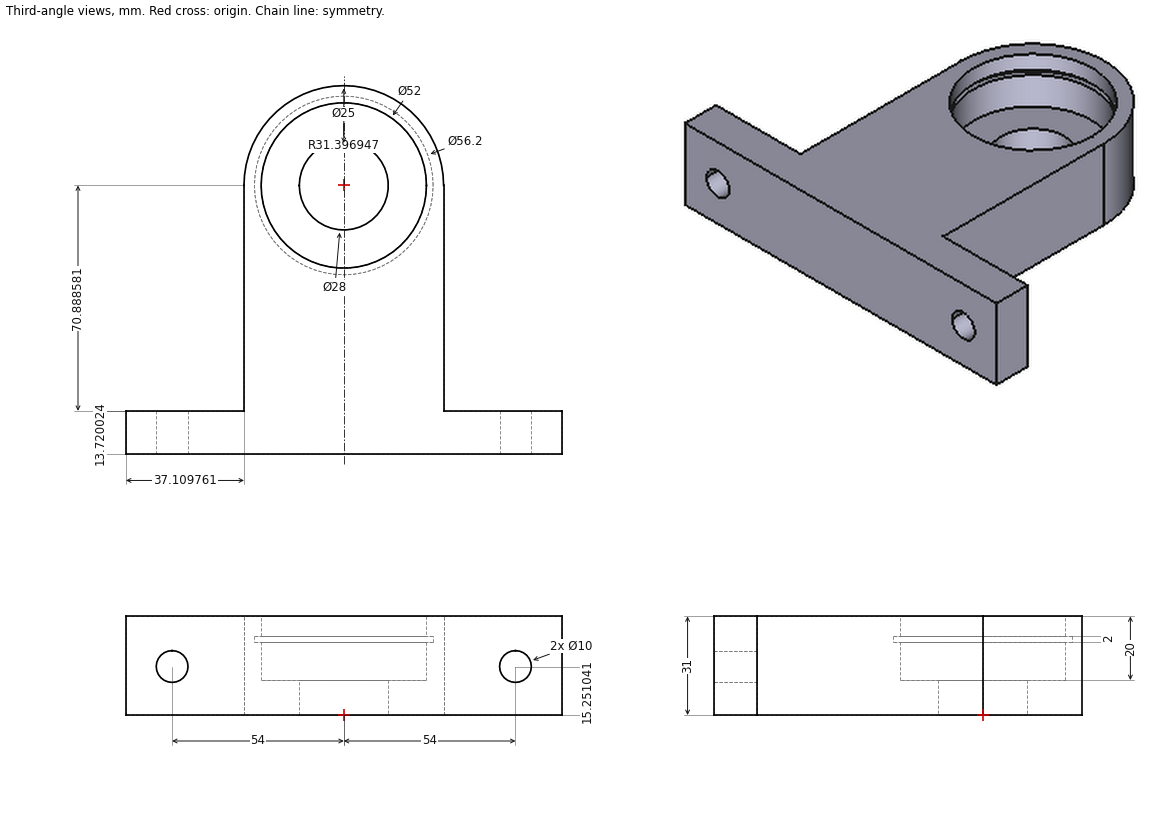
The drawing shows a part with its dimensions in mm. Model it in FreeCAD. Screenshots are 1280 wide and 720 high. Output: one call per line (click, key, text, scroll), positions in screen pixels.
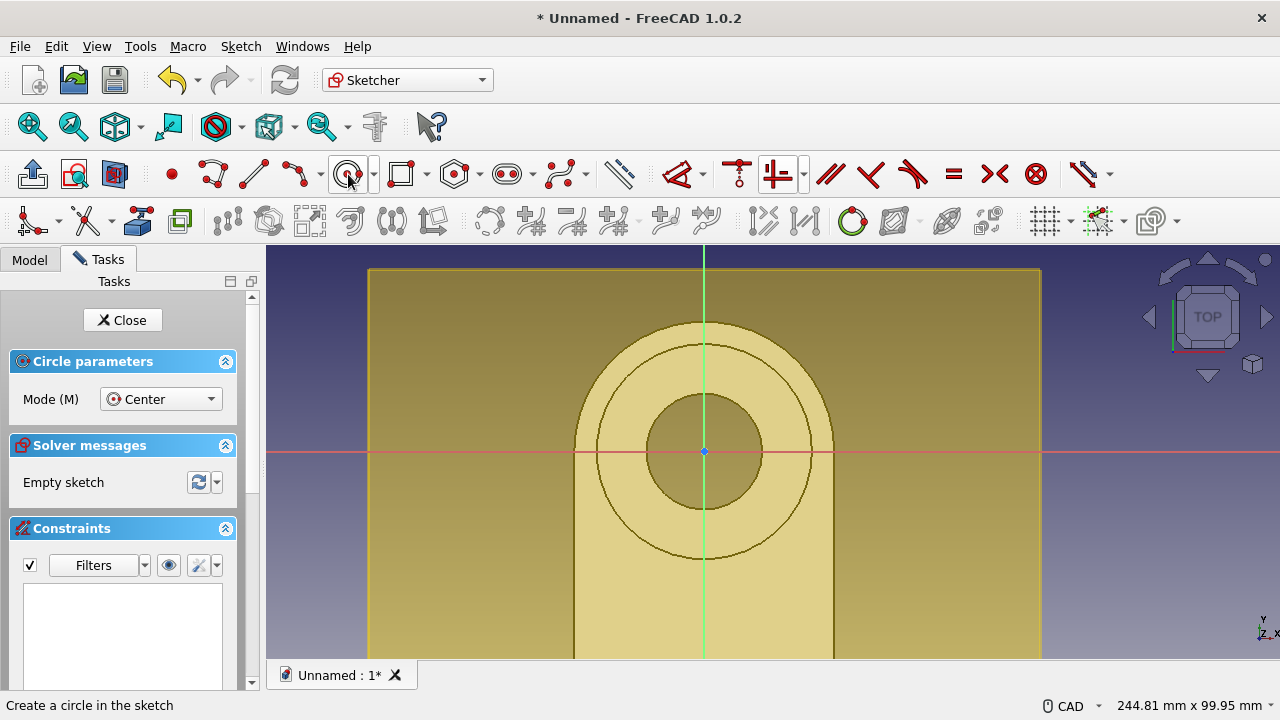
click(704, 452)
click(787, 369)
key(Escape)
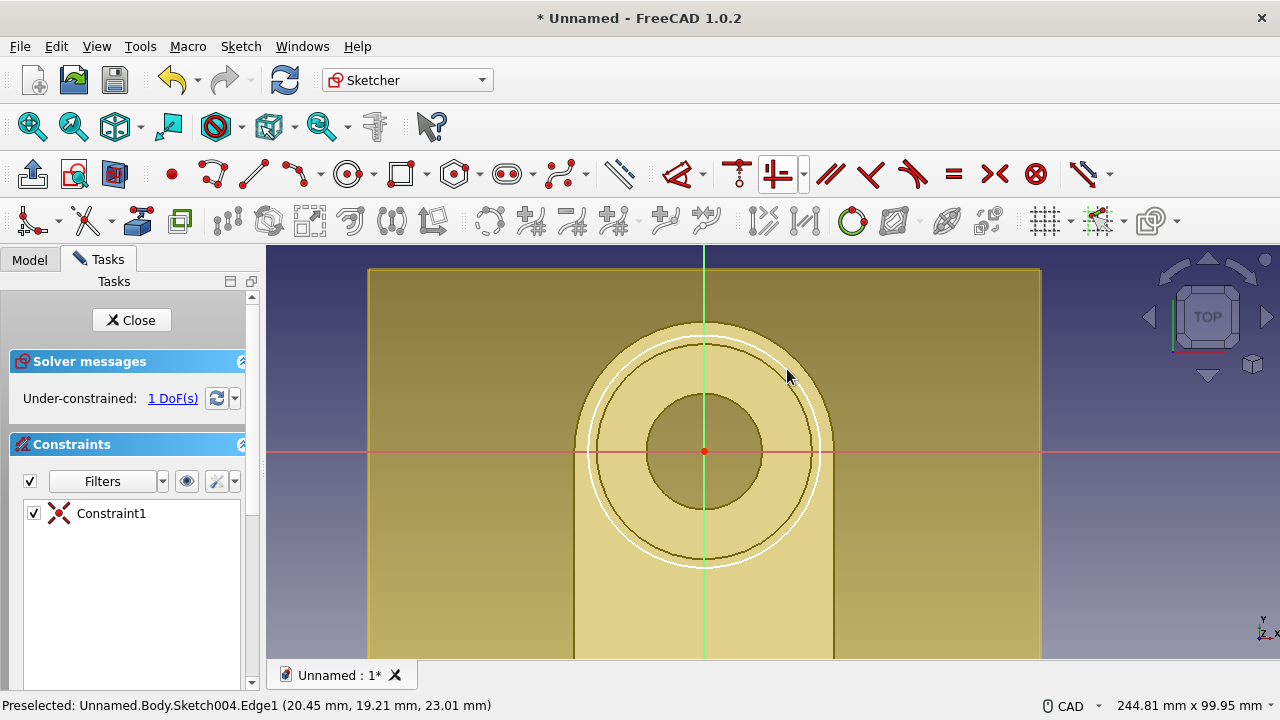
key(d)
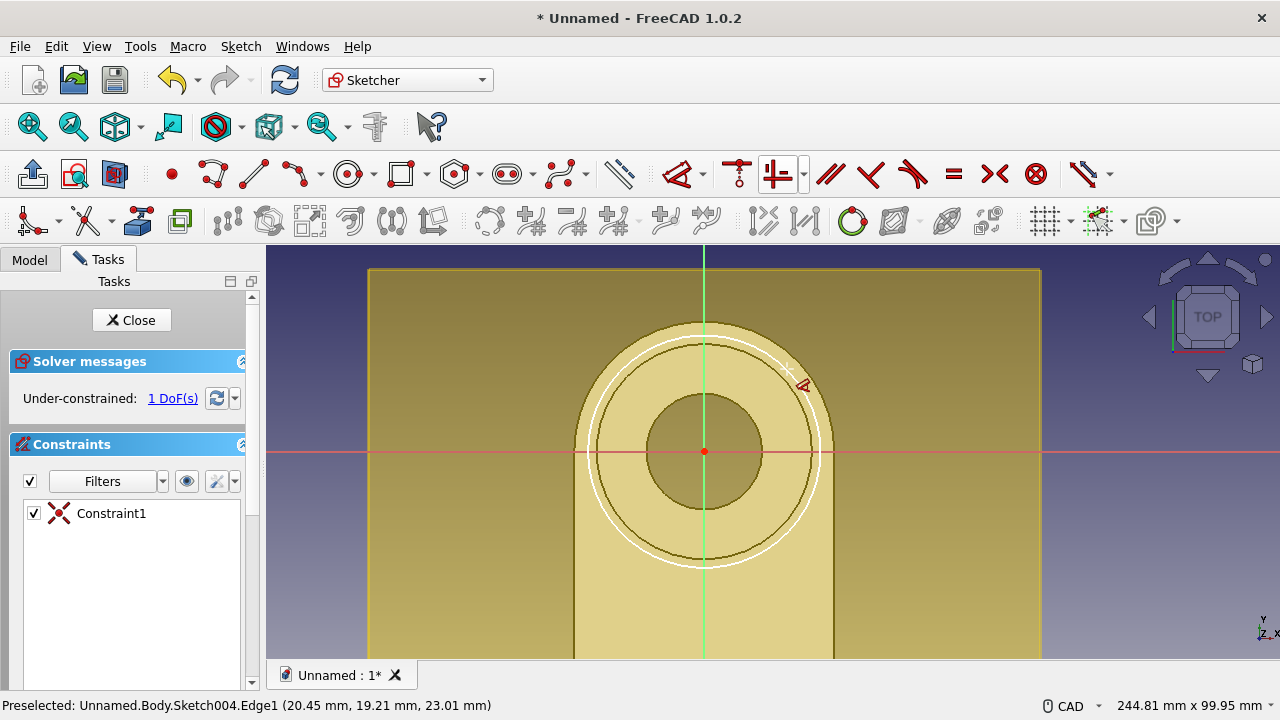
click(786, 369)
click(808, 346)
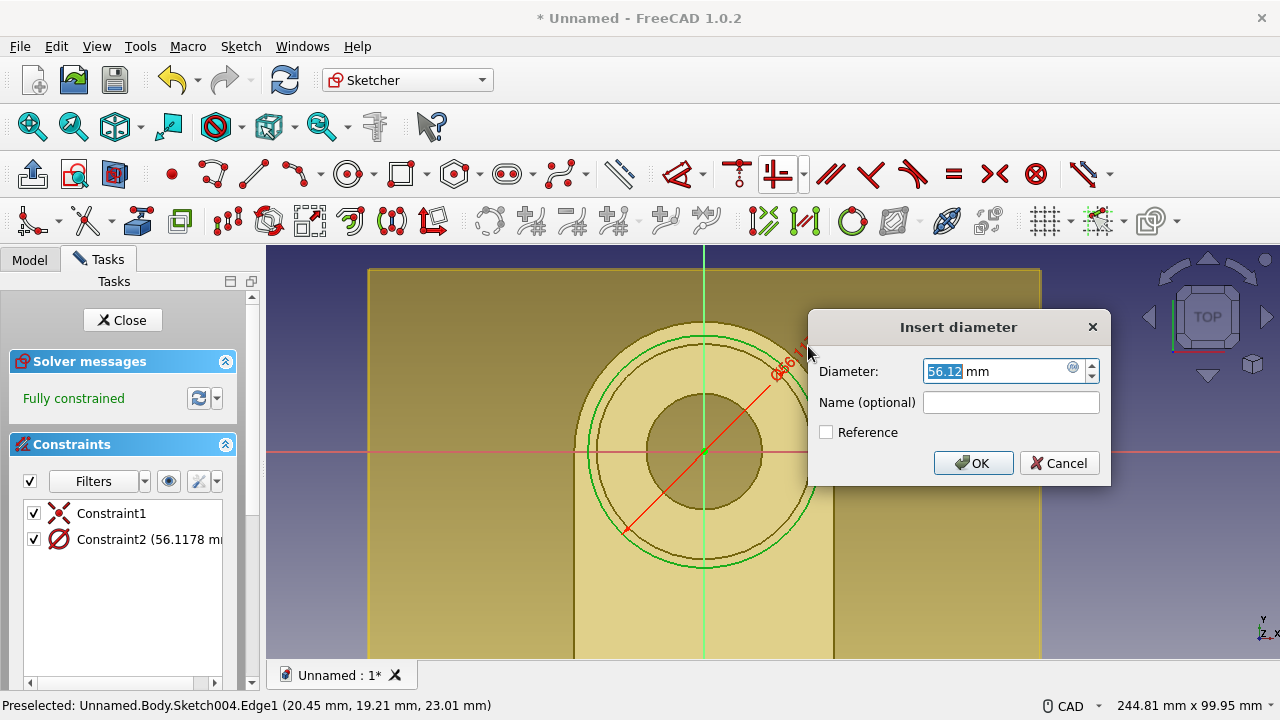
text(56.2)
key(Return)
key(Escape)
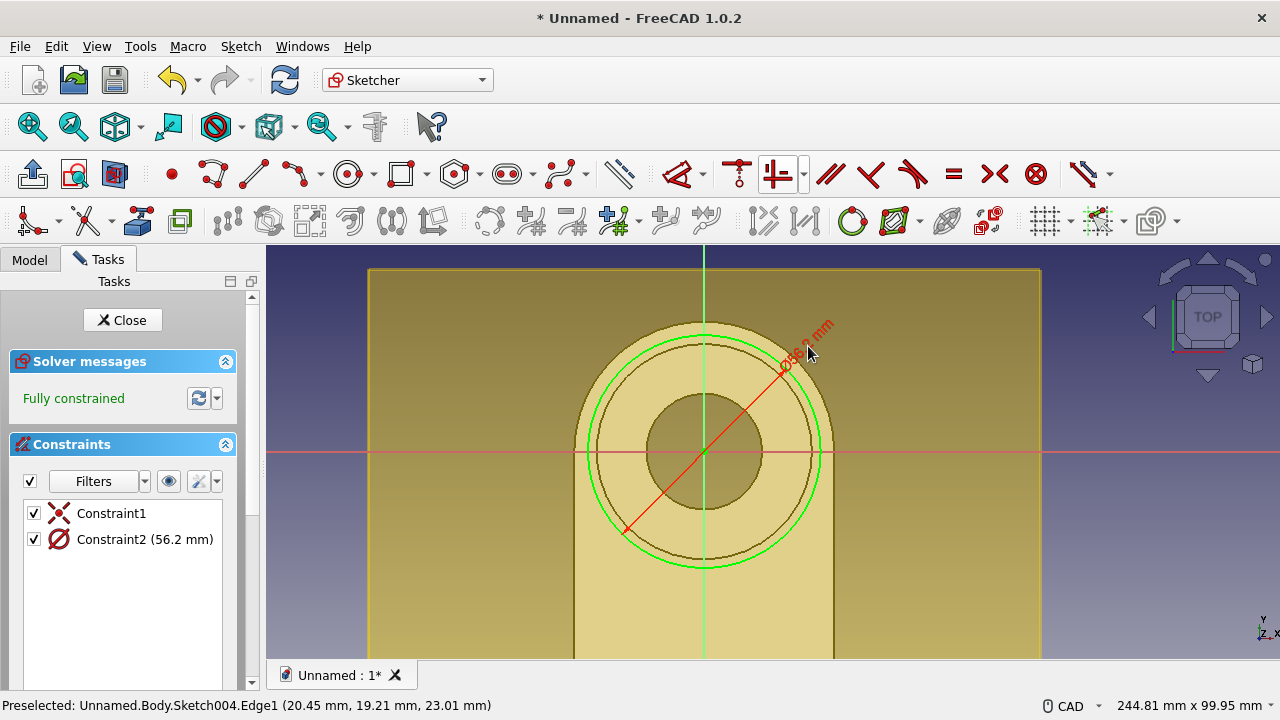
click(123, 320)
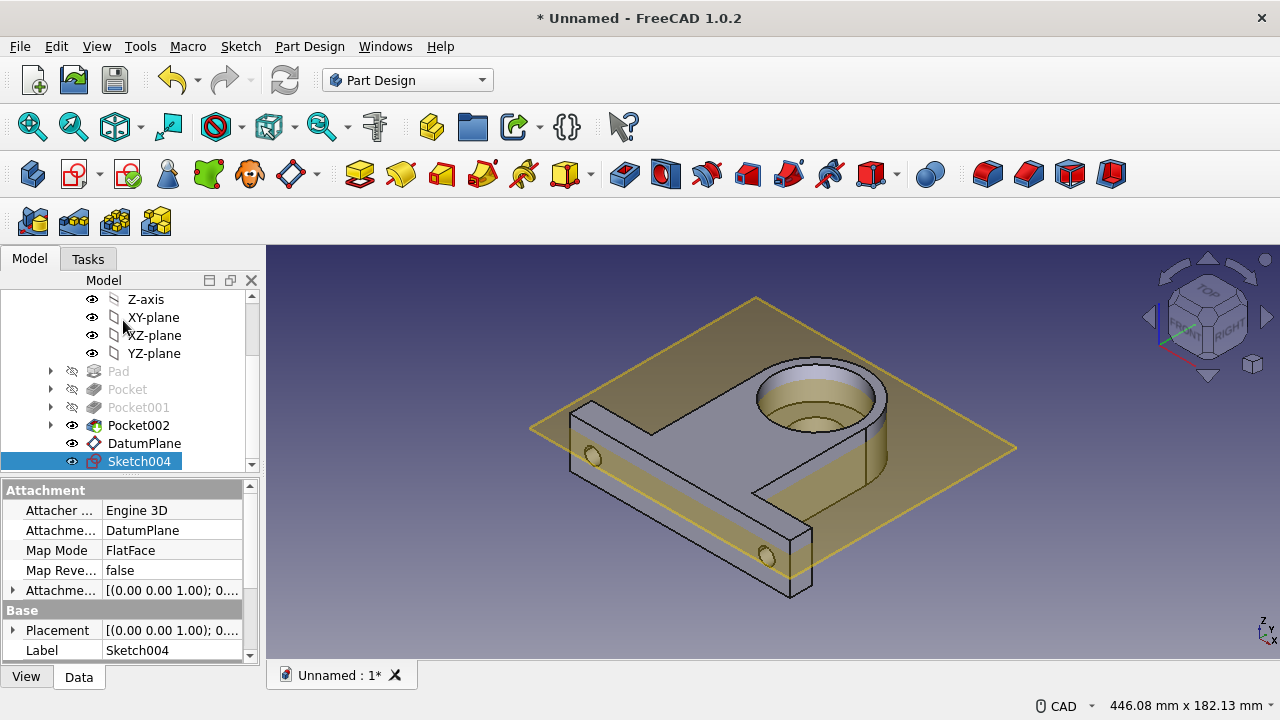
click(625, 174)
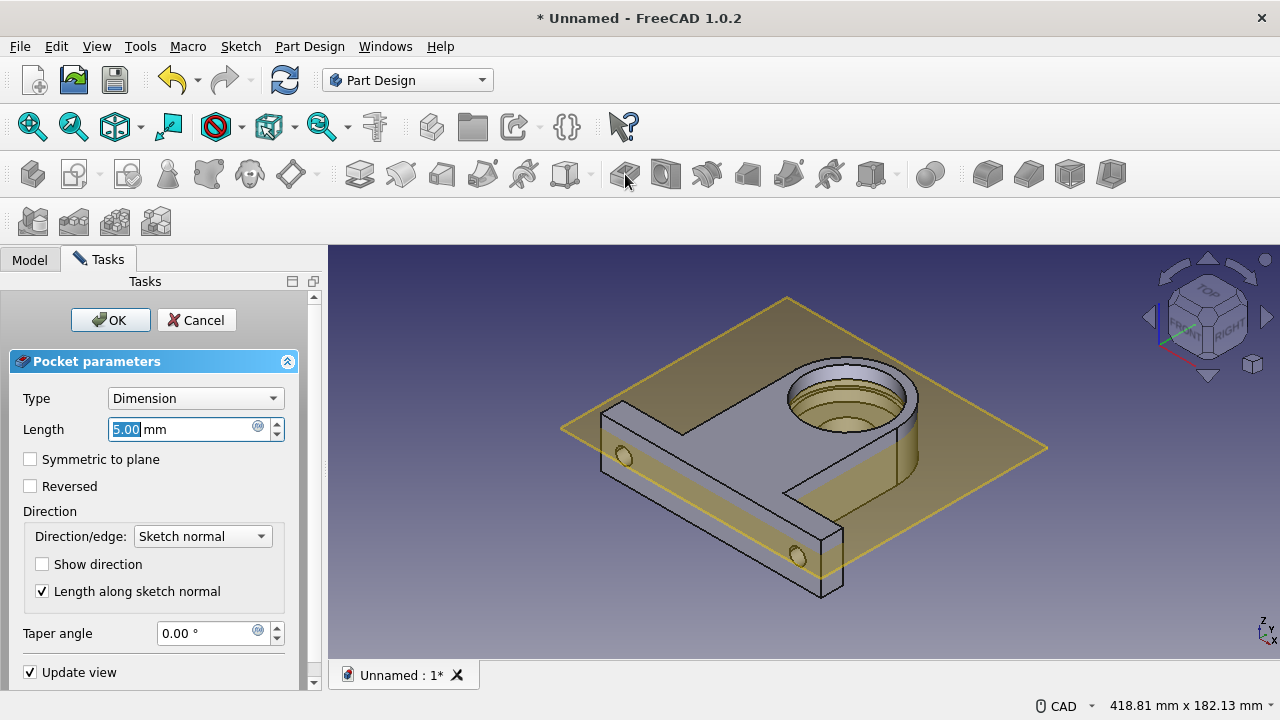
text(2)
key(Tab)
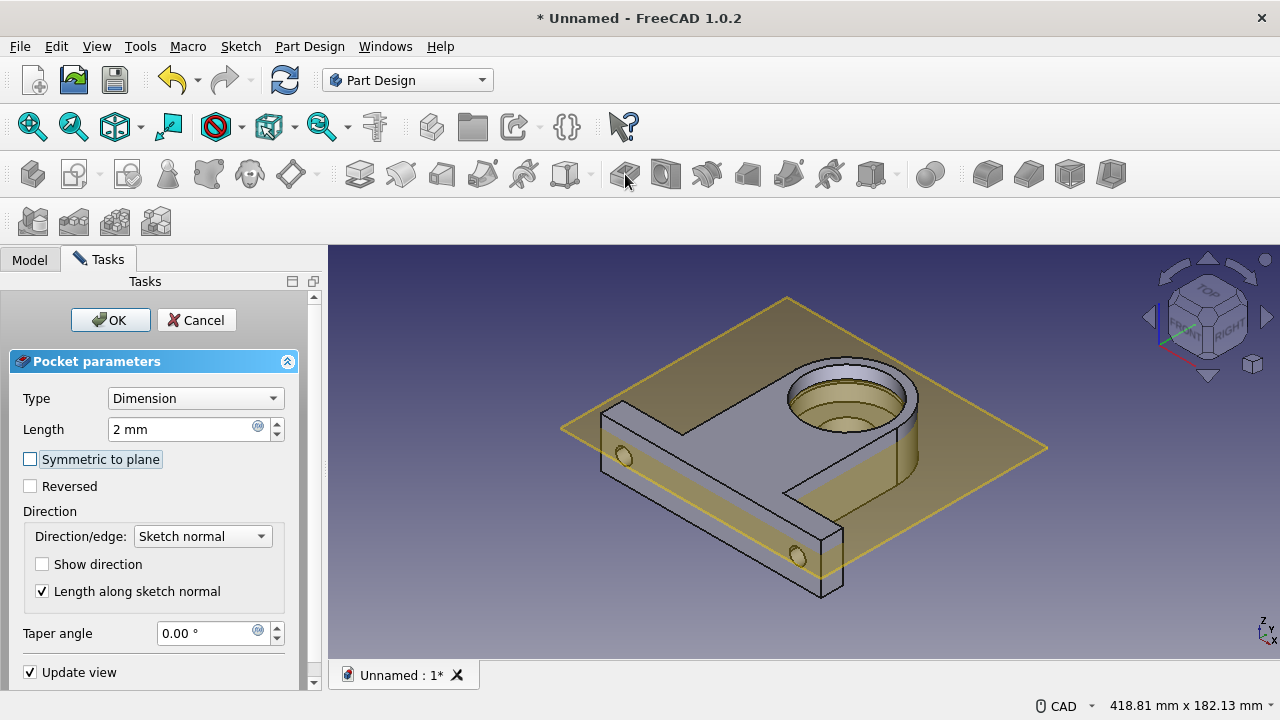
click(31, 486)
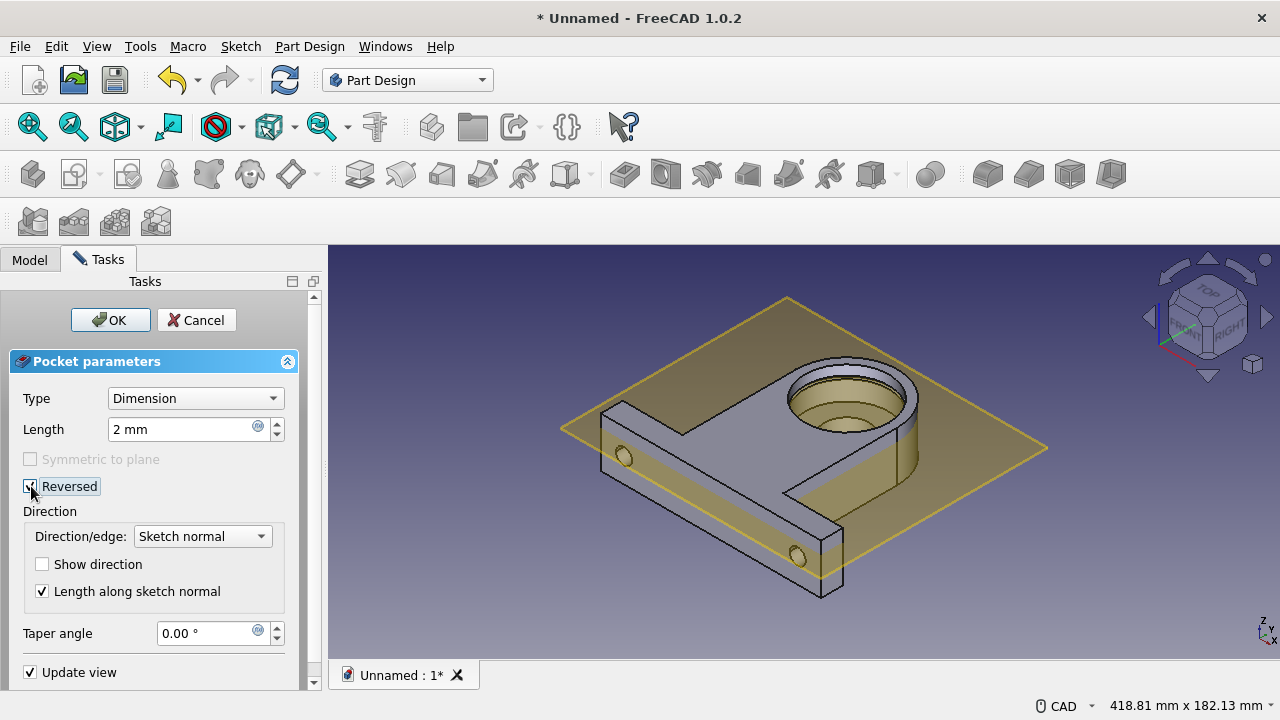
click(111, 320)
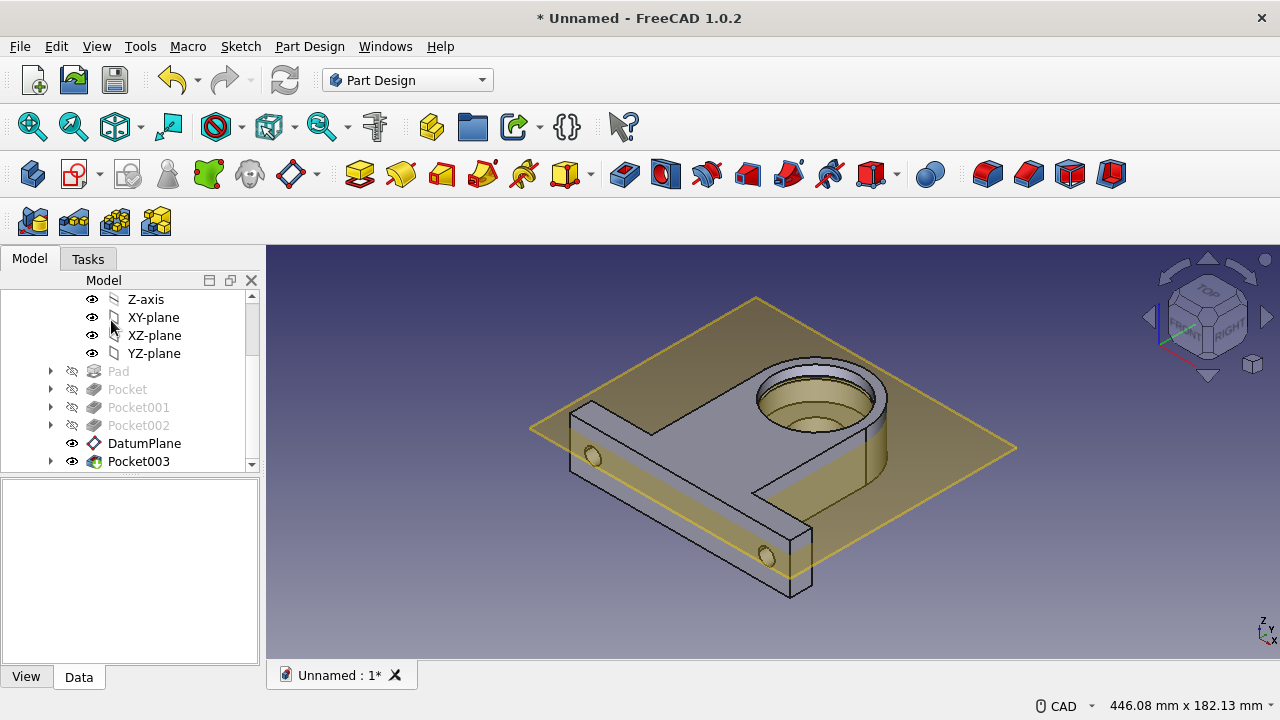
click(117, 443)
key(space)